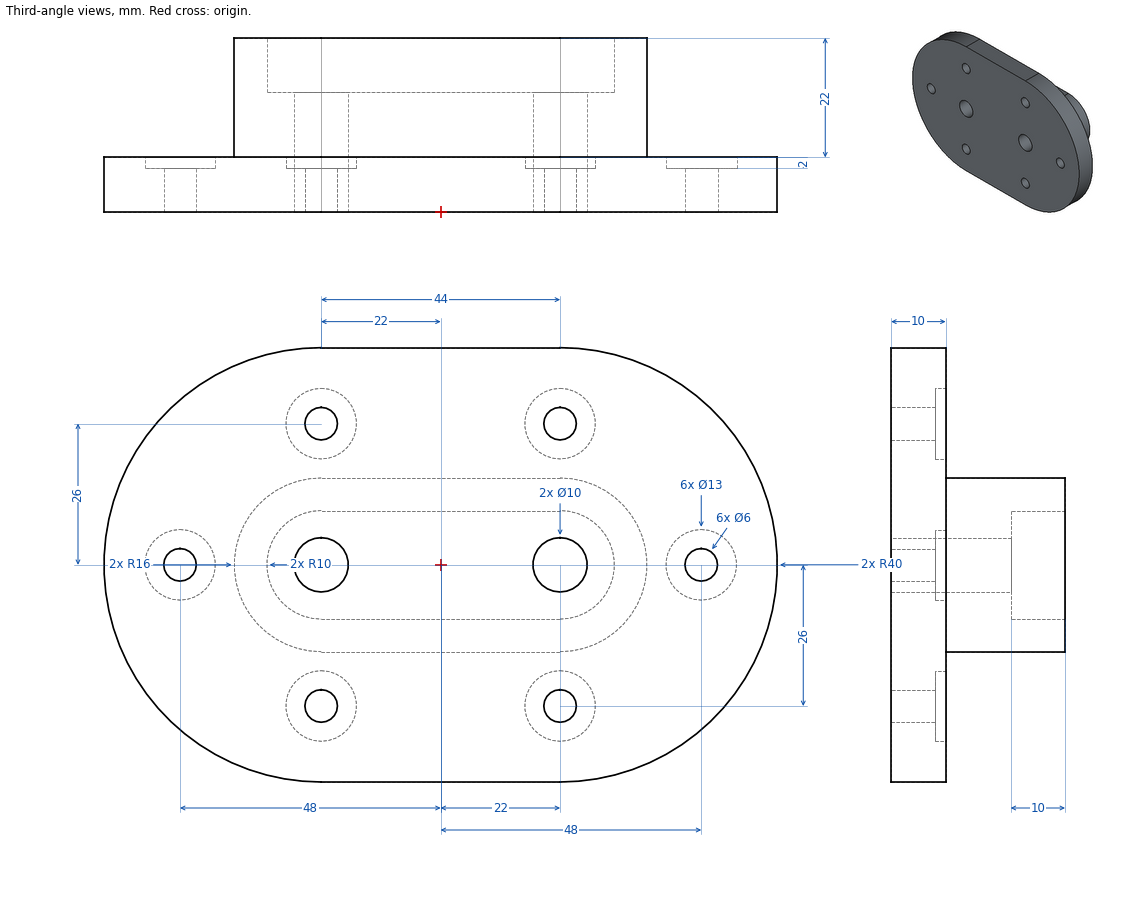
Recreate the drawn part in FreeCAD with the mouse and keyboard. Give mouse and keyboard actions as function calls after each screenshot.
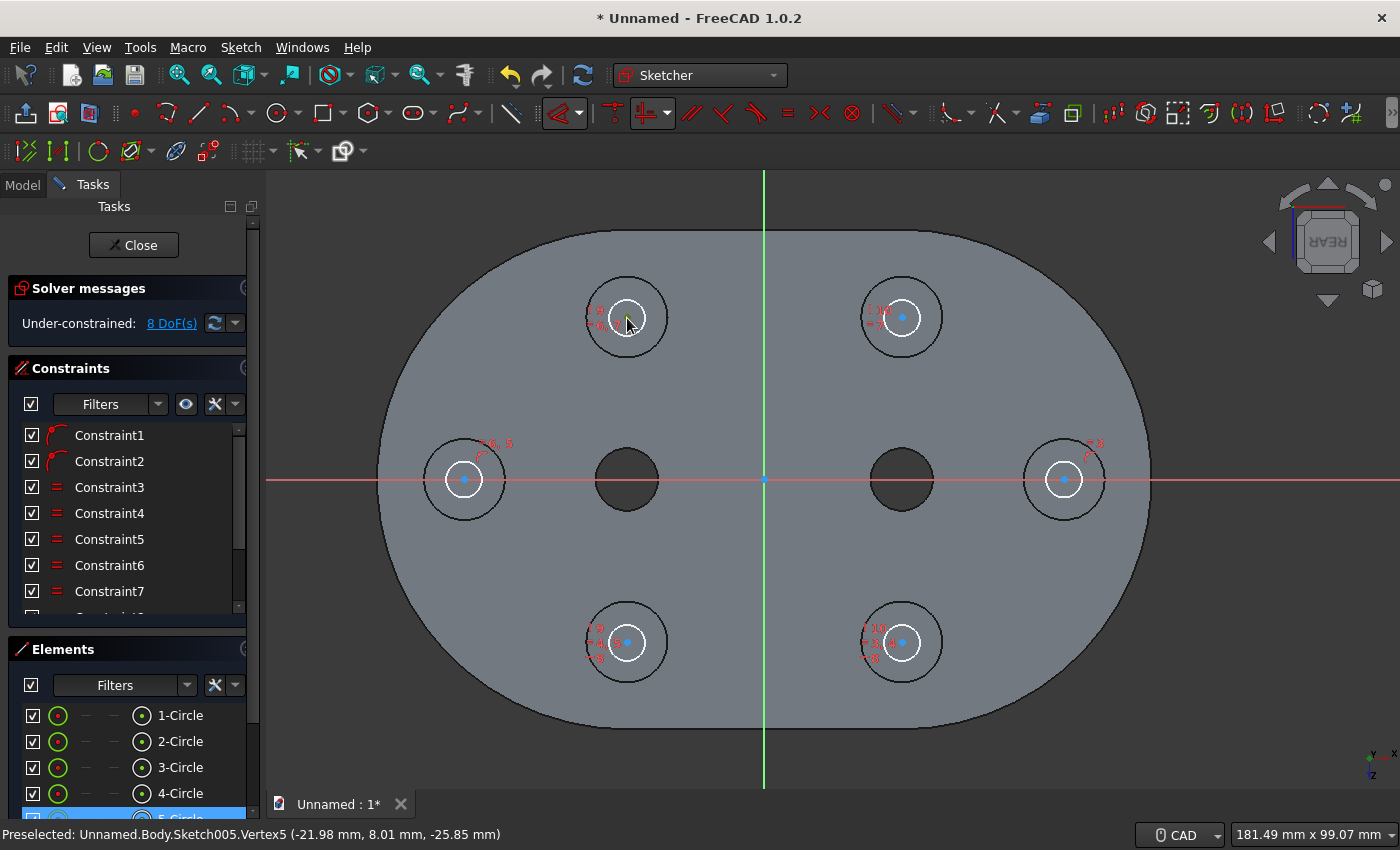
click(902, 318)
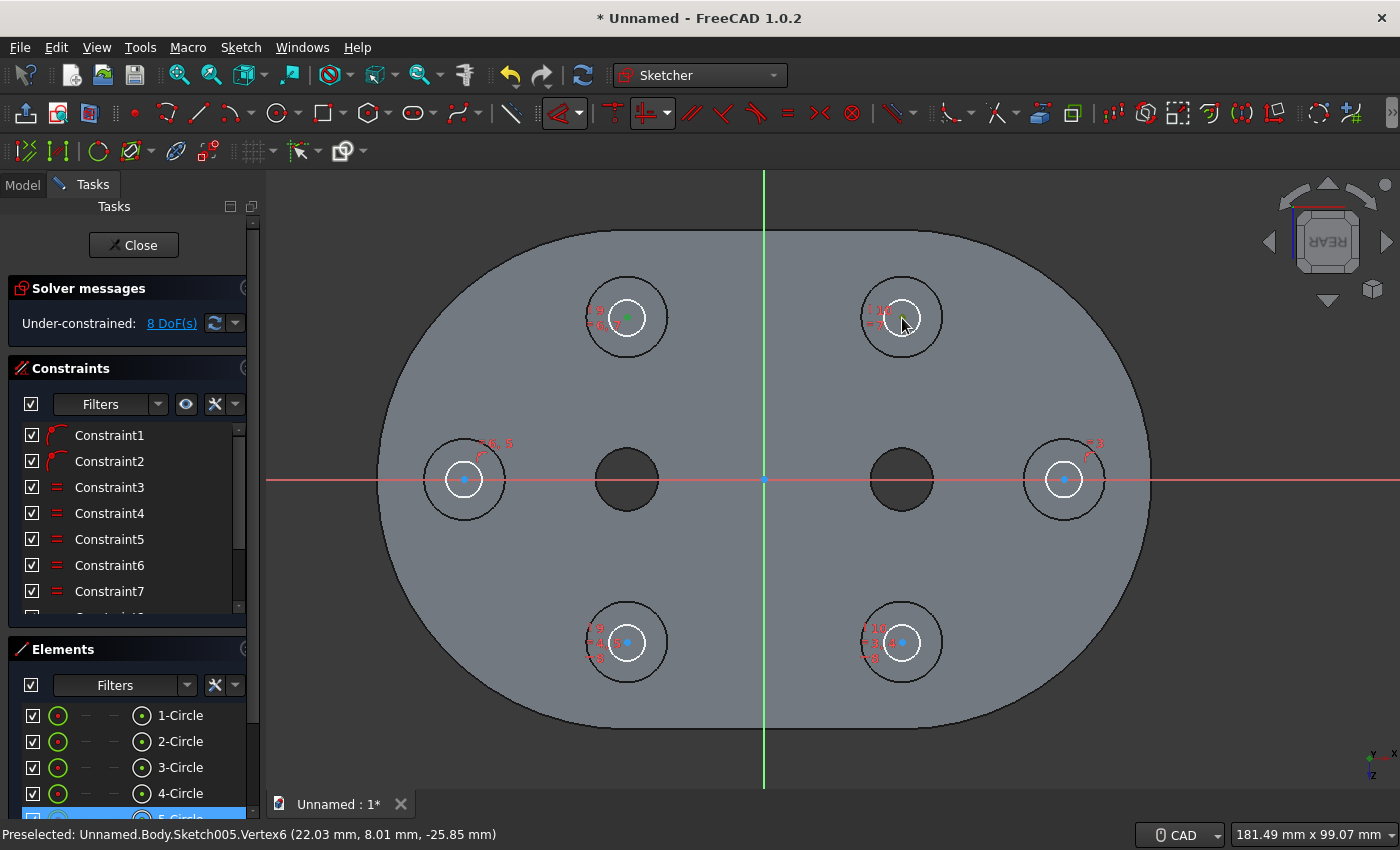
click(670, 114)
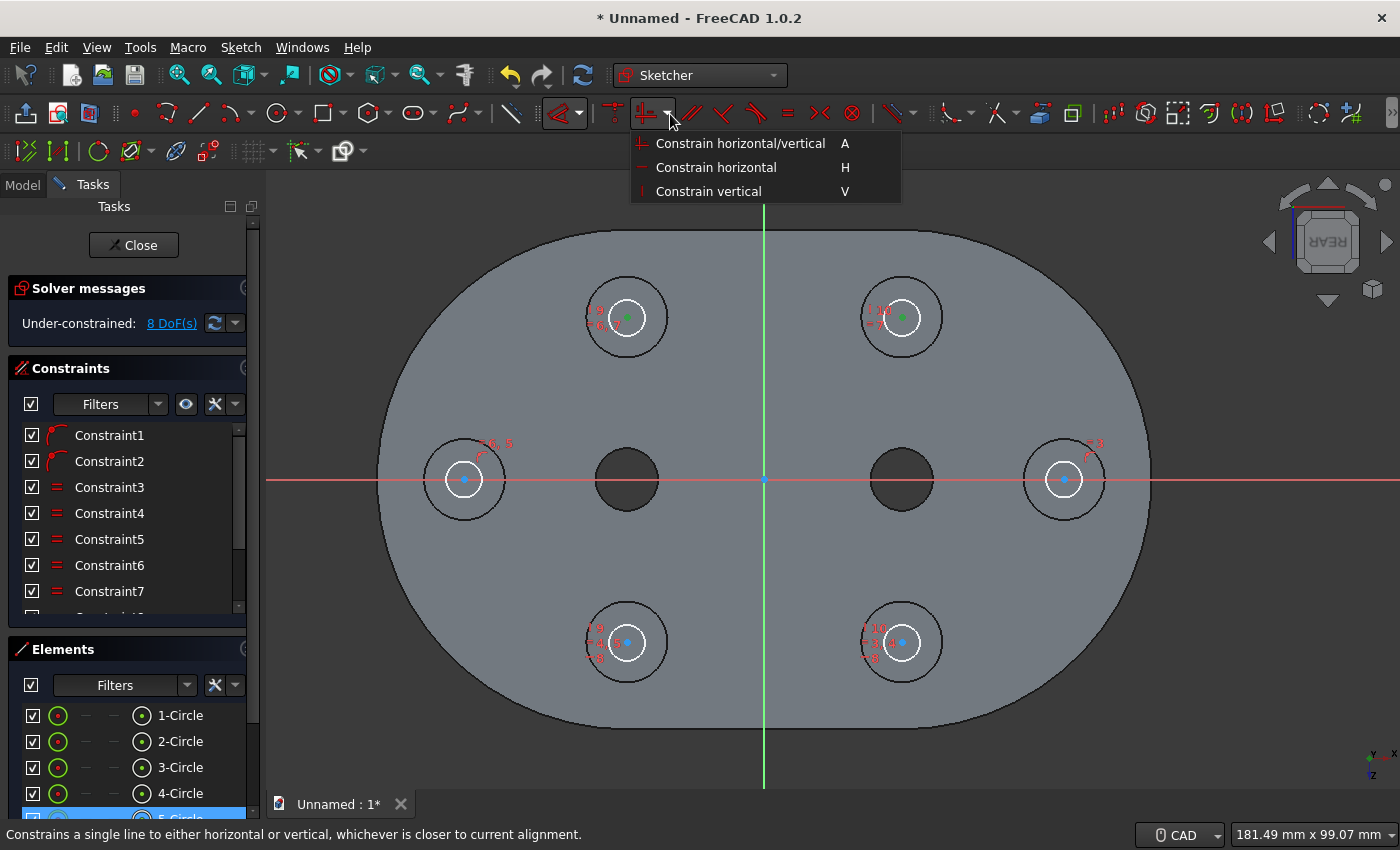
click(766, 167)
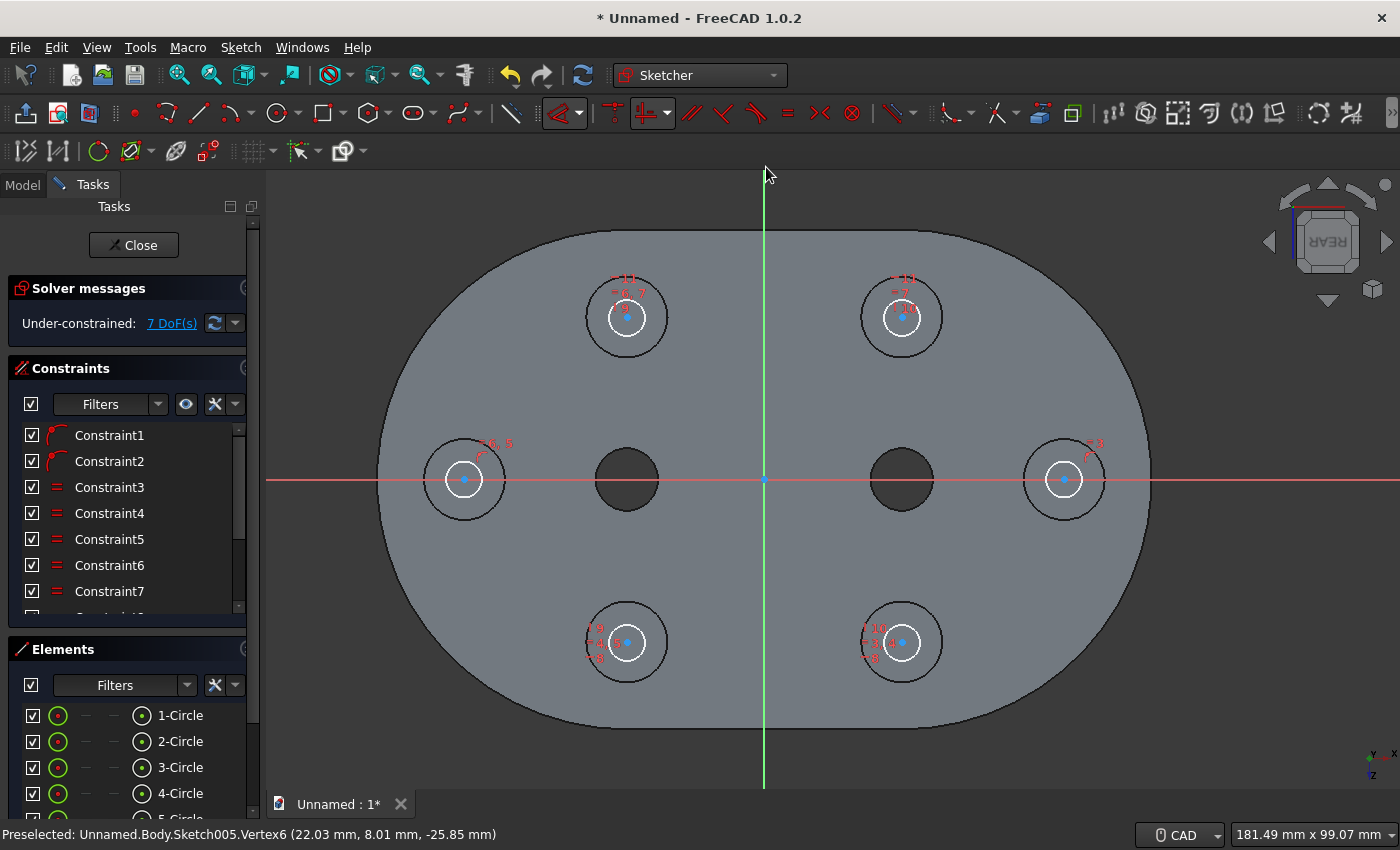
click(1077, 467)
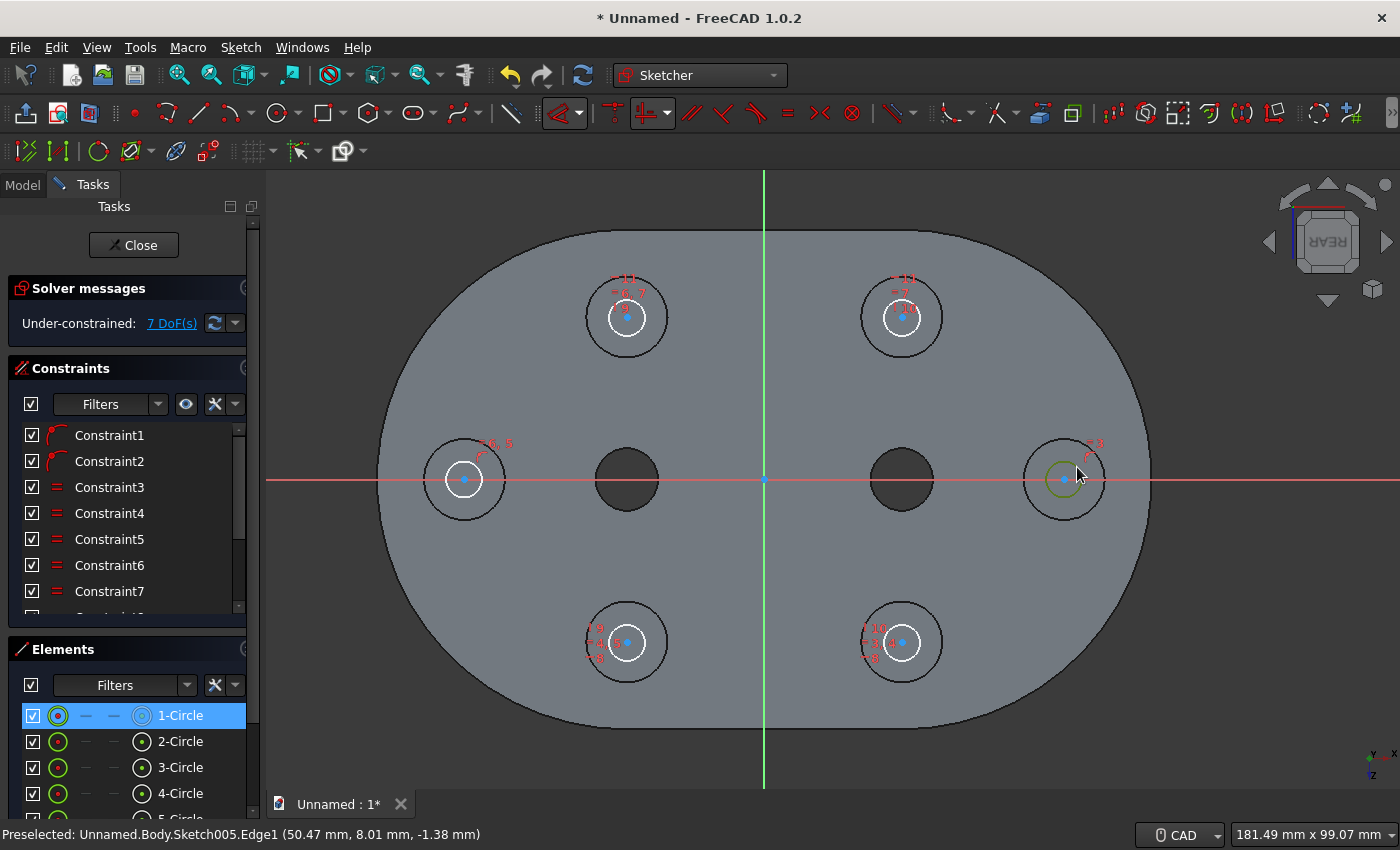
key(k)
key(o)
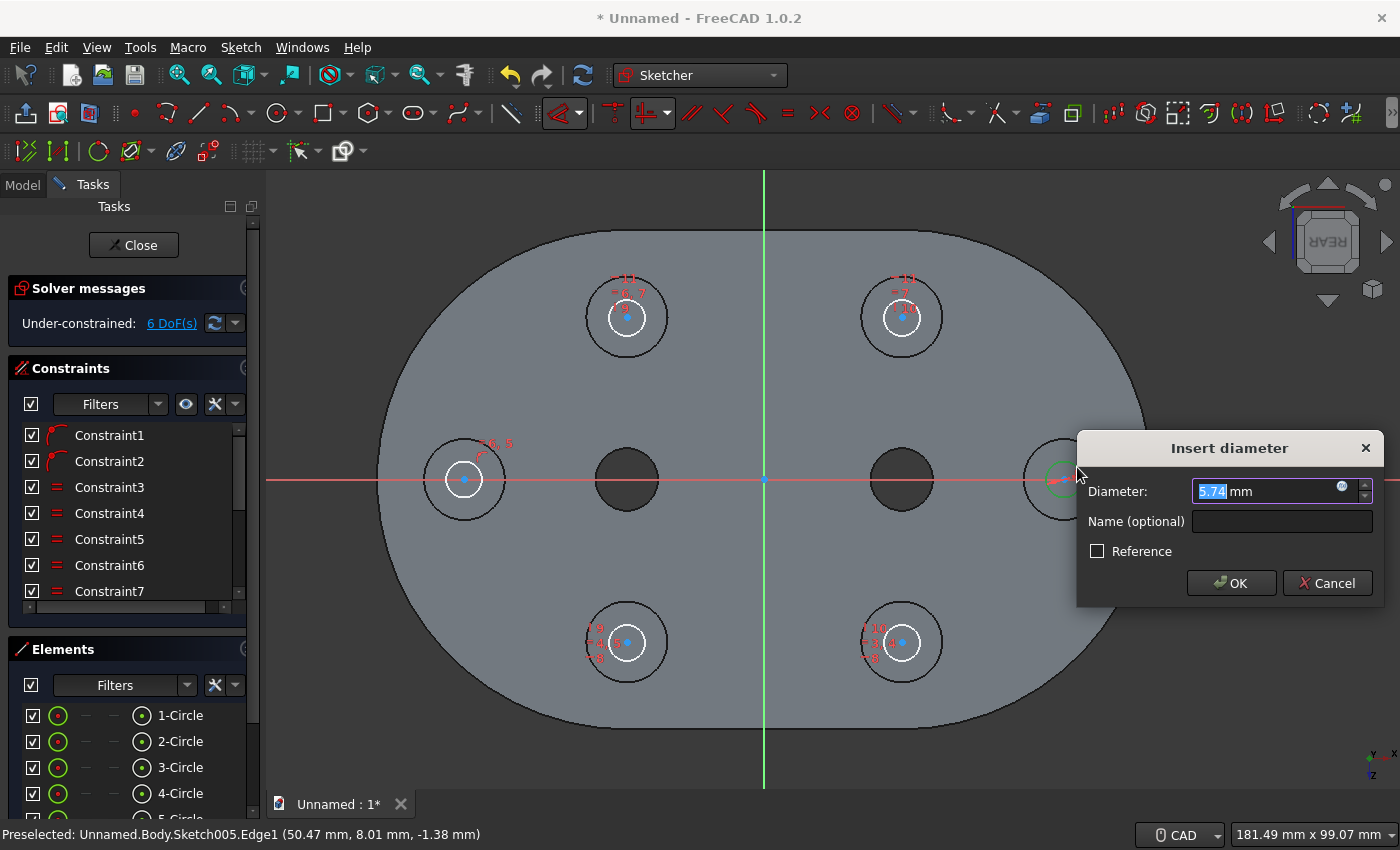
text(6)
key(Return)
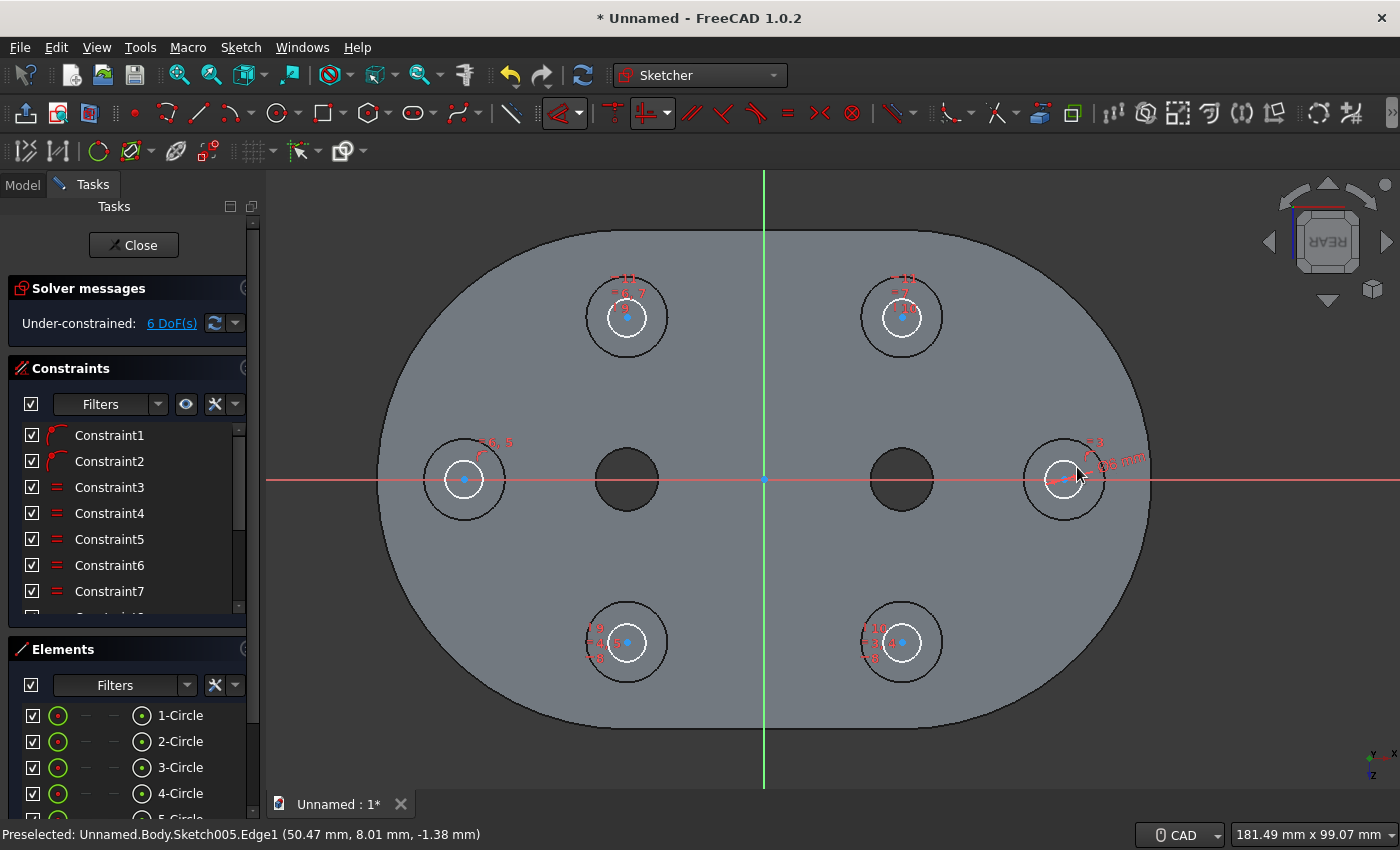
click(1064, 479)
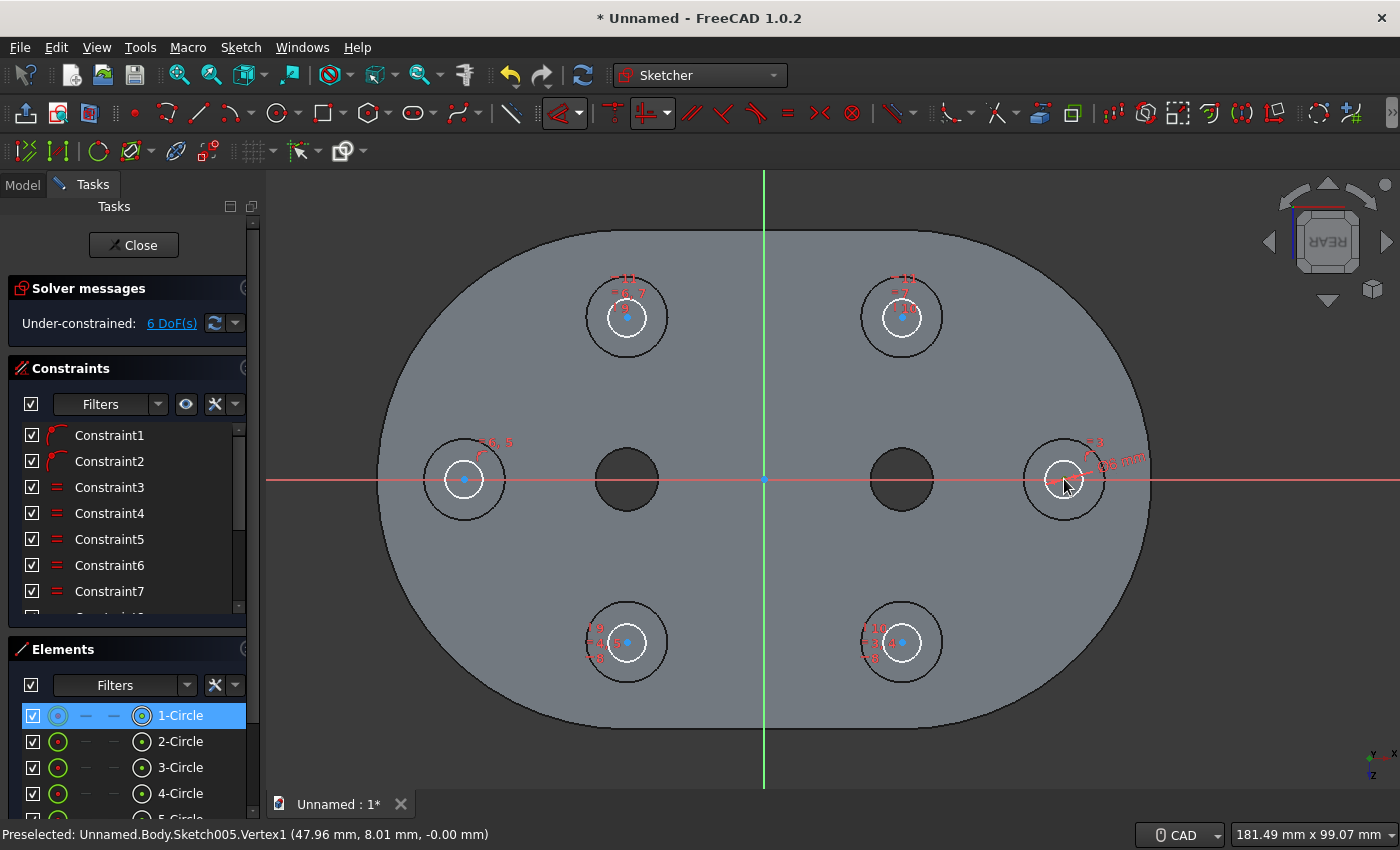
key(l)